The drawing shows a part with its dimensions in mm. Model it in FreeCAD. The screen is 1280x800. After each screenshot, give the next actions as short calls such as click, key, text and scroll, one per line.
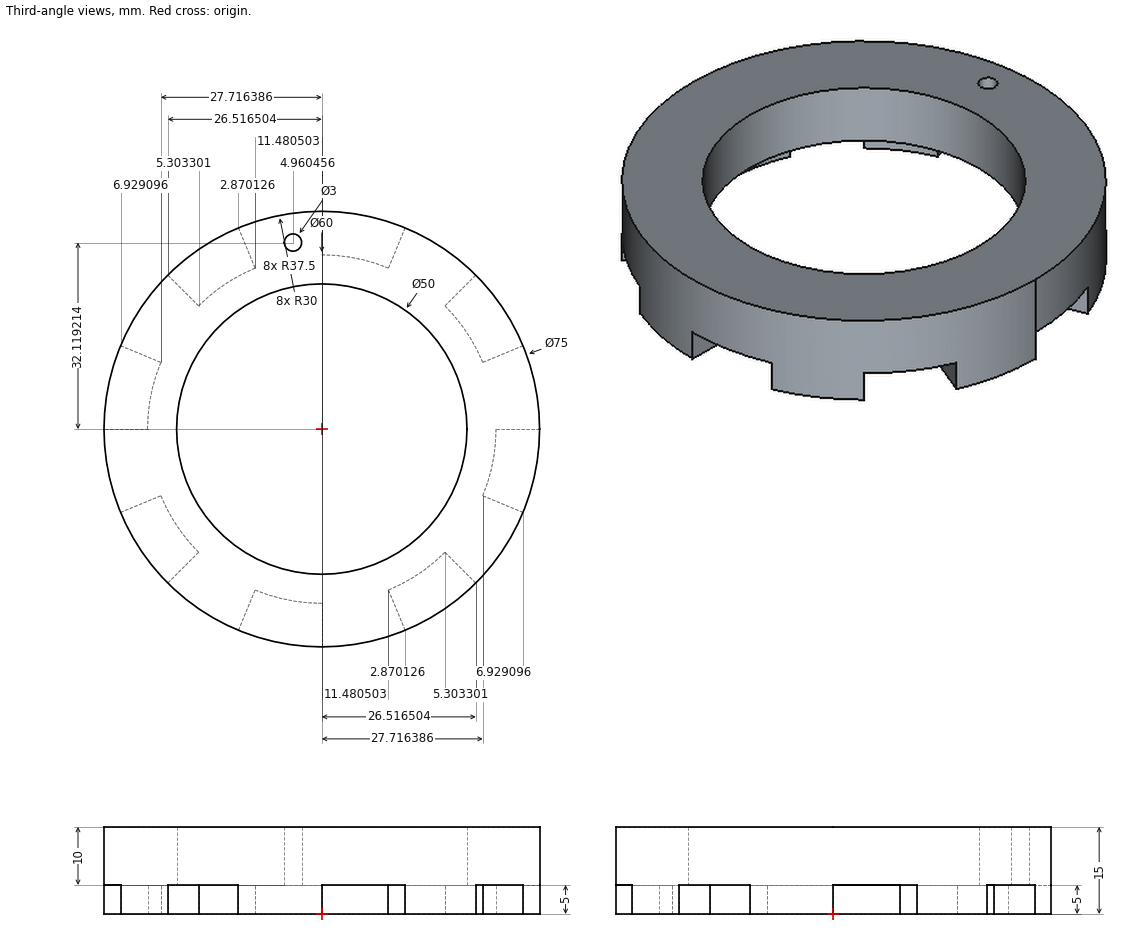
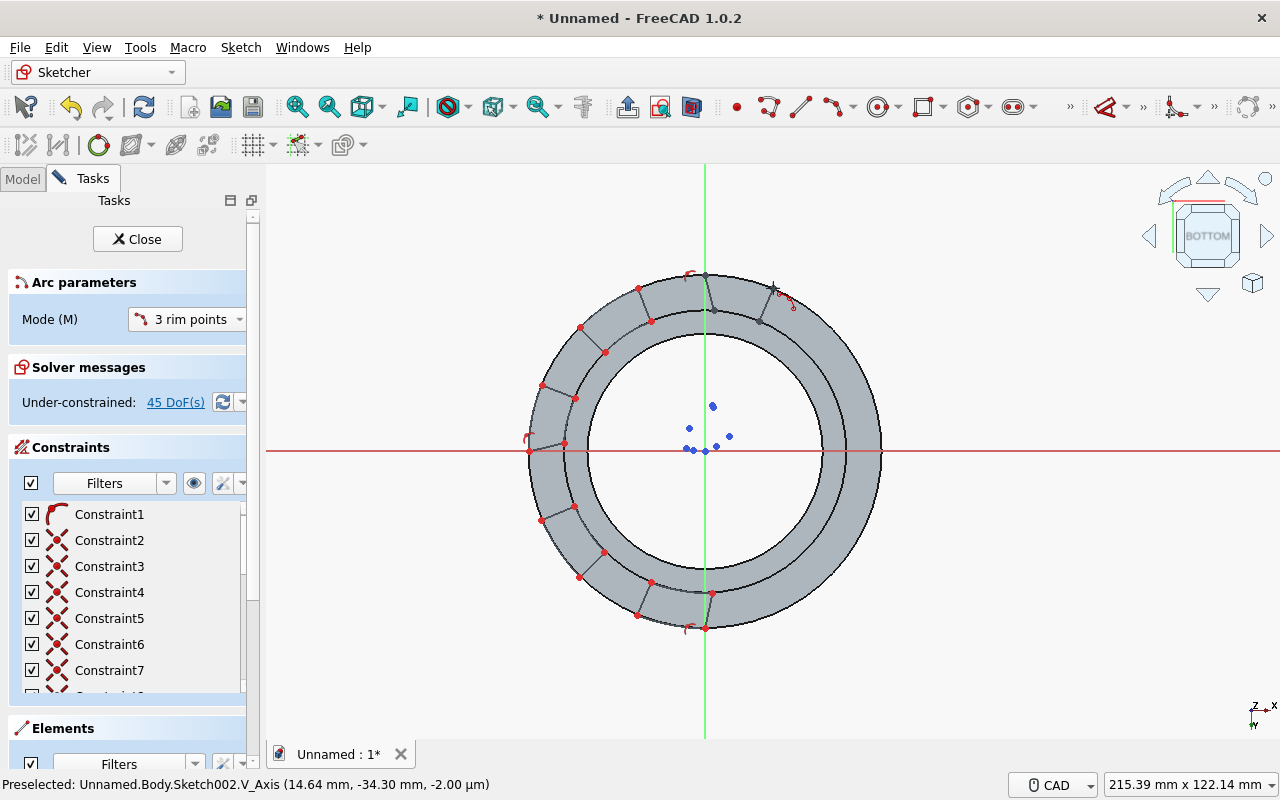
click(714, 311)
click(759, 322)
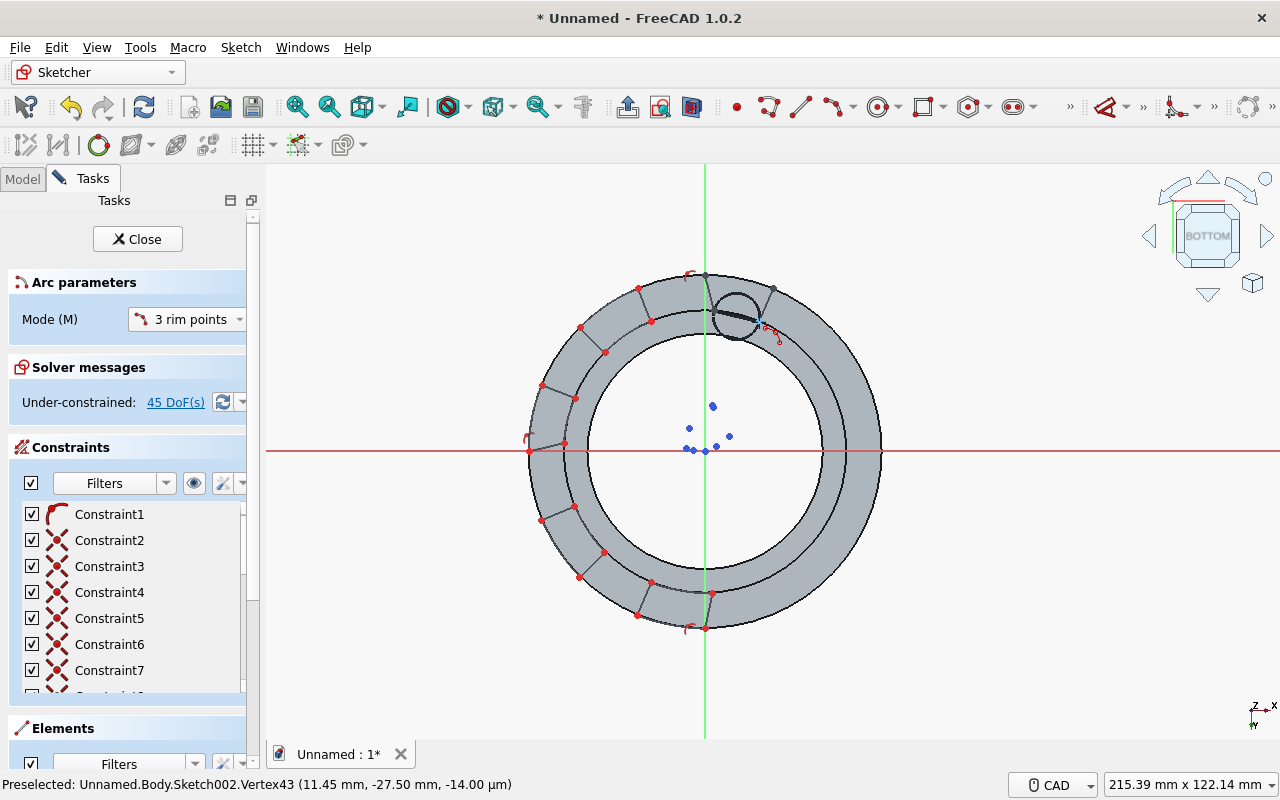
scroll(733, 313, up, 9)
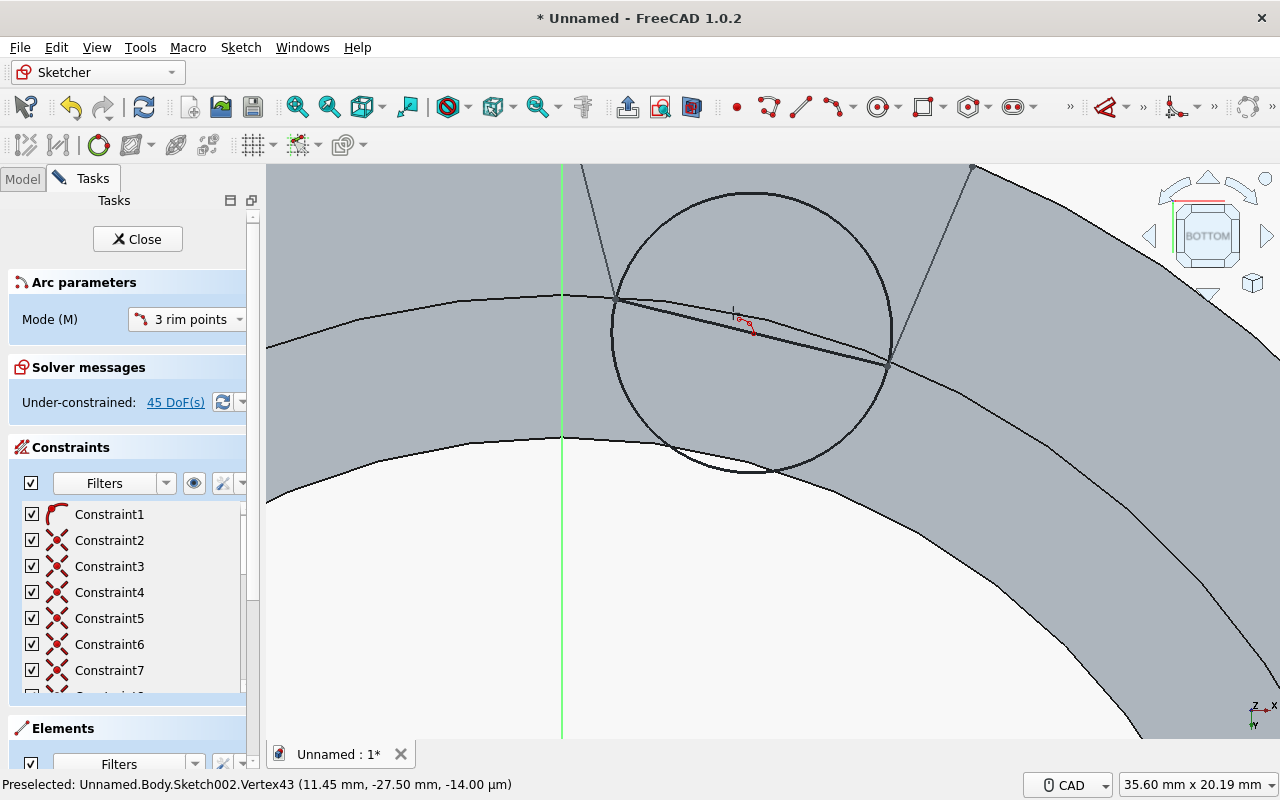
click(729, 311)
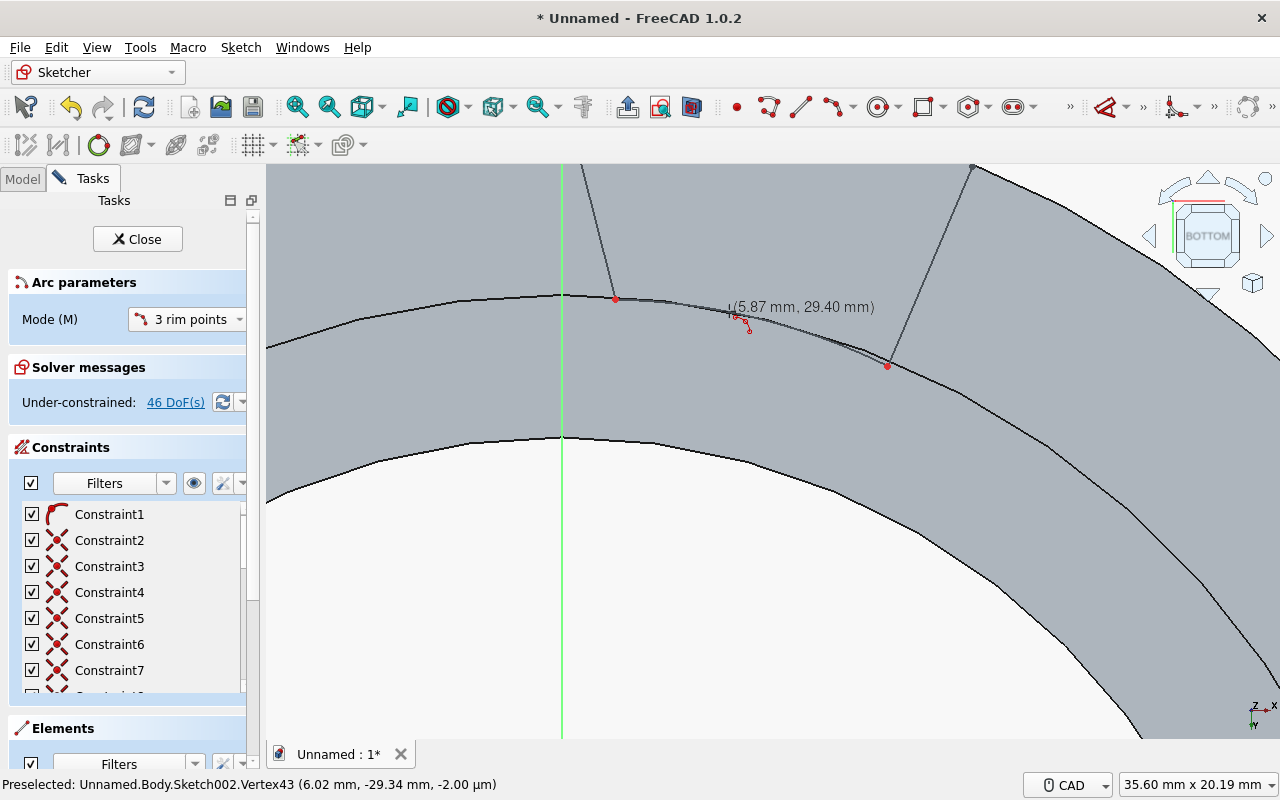
scroll(733, 313, down, 9)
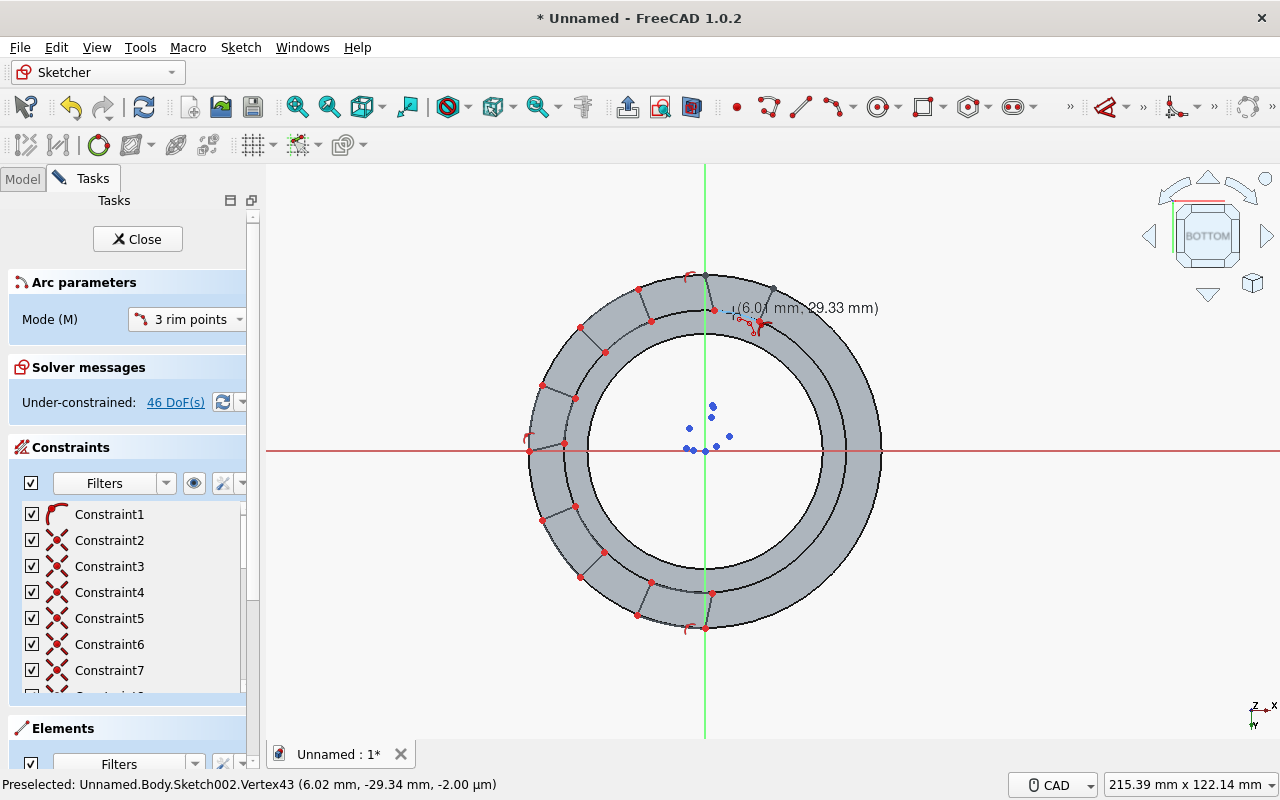
click(773, 289)
click(705, 276)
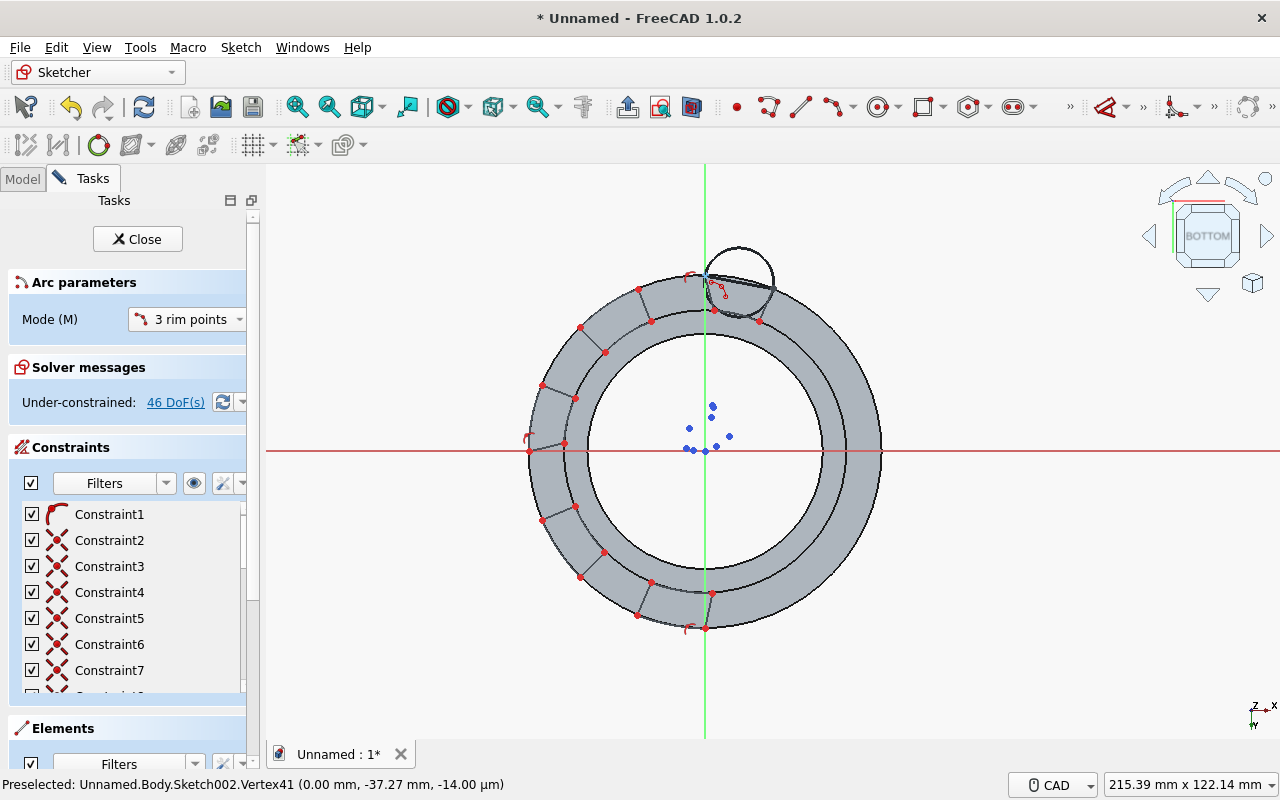
scroll(740, 278, up, 8)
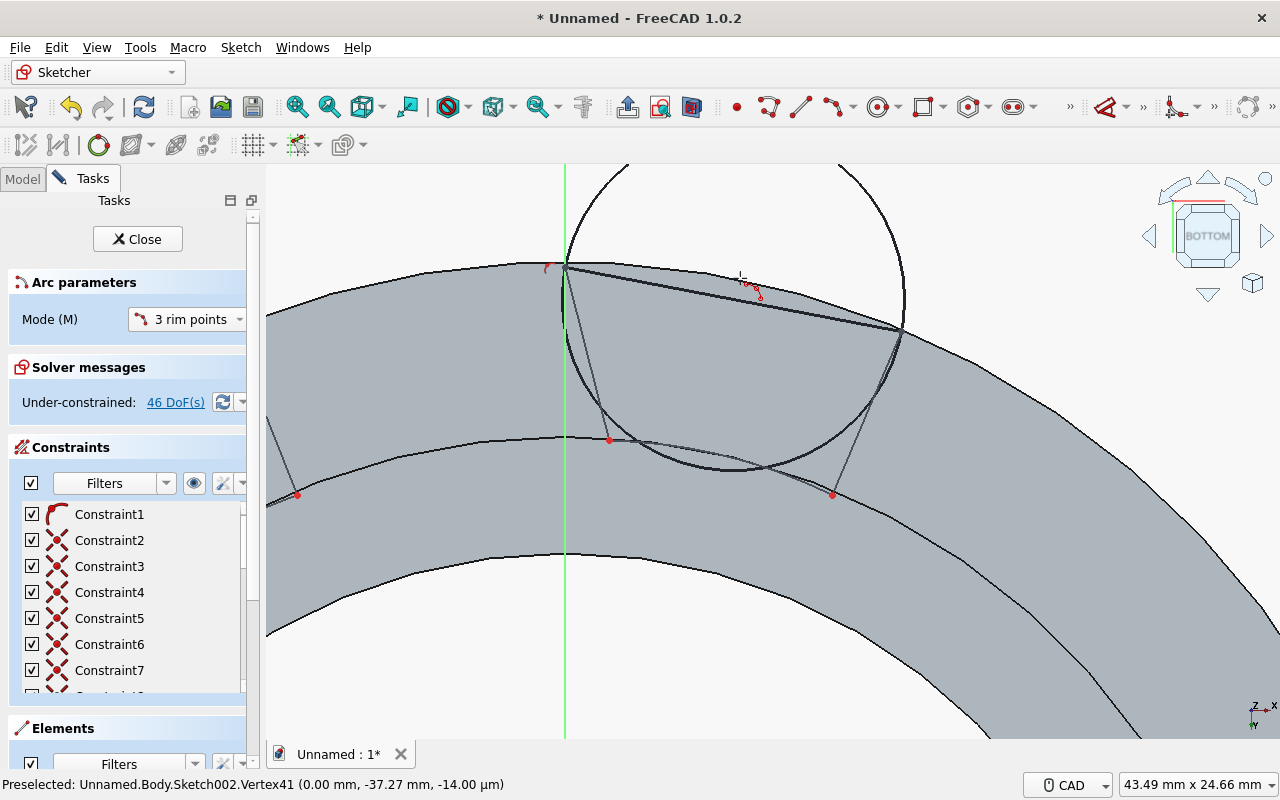
click(736, 279)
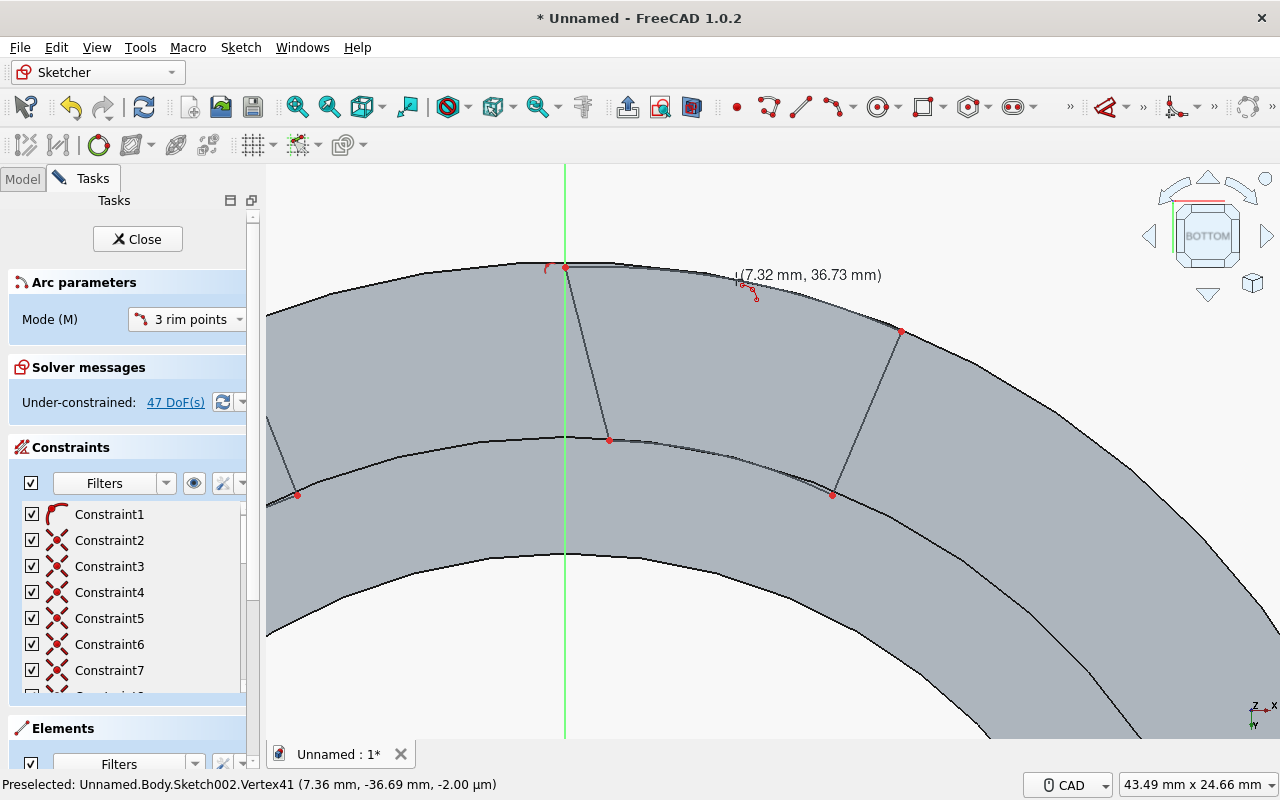
key(g)
key(l)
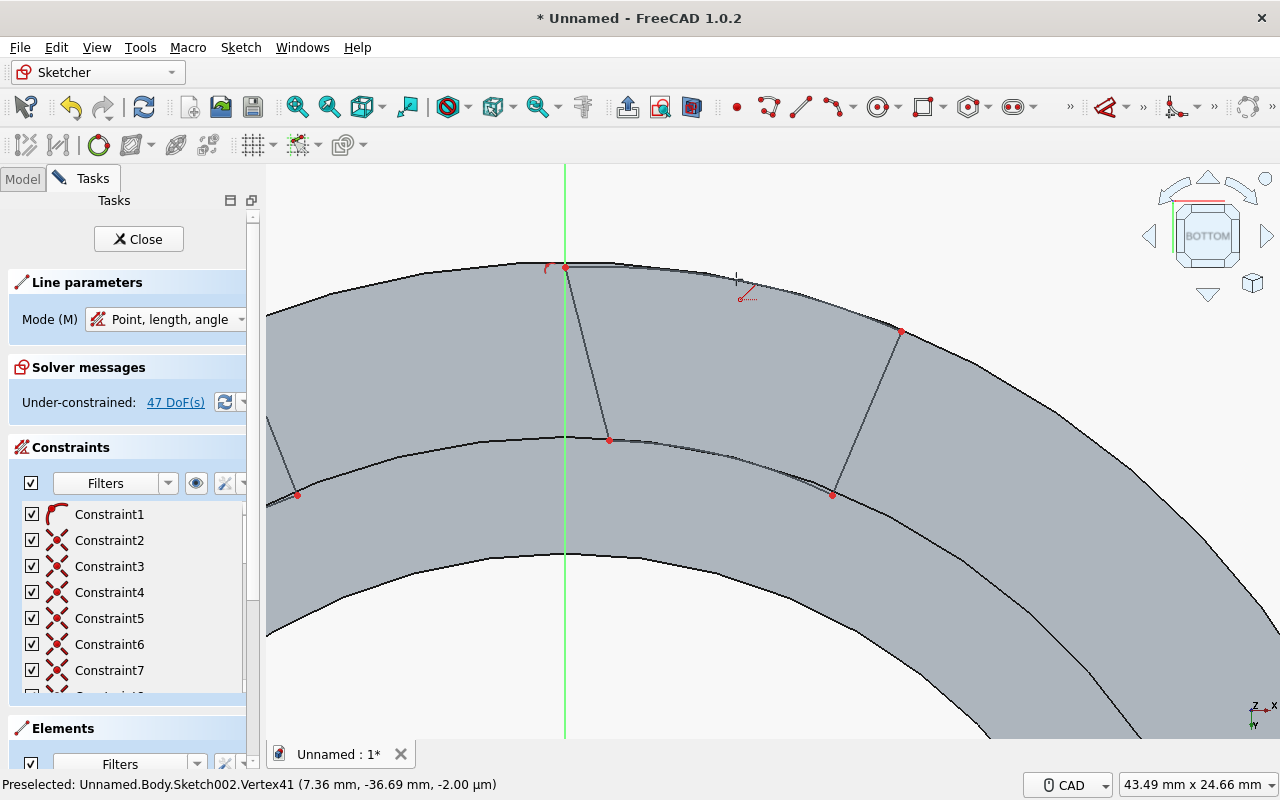
scroll(740, 278, down, 8)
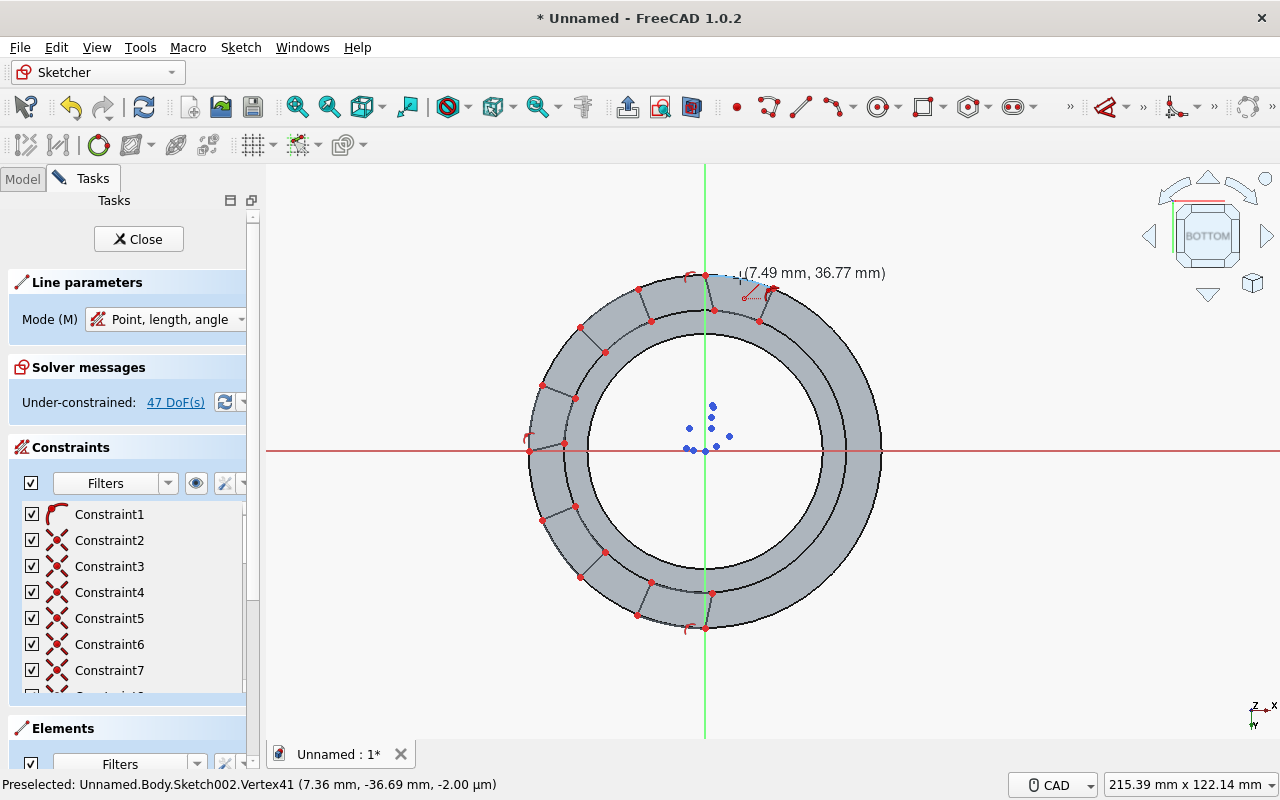
click(830, 327)
click(805, 352)